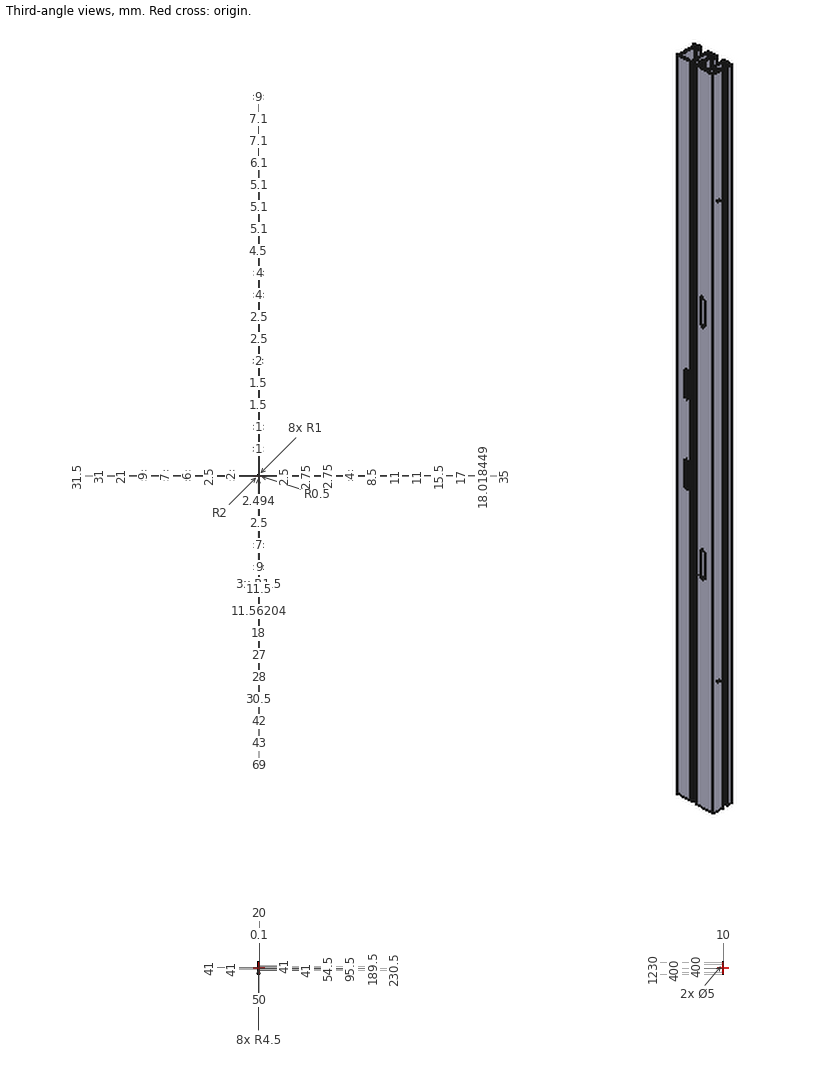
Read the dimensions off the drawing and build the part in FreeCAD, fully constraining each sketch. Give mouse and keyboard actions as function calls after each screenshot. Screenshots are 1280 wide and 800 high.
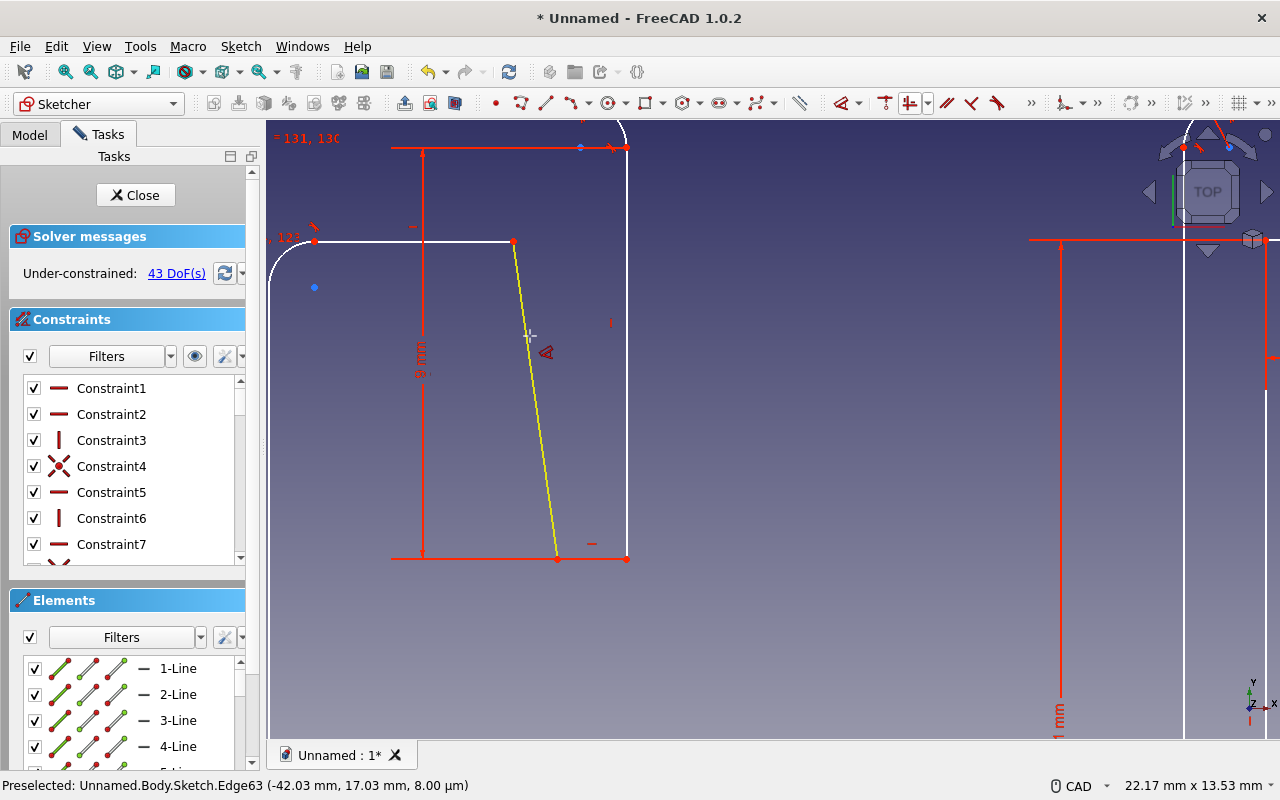
click(526, 337)
click(535, 208)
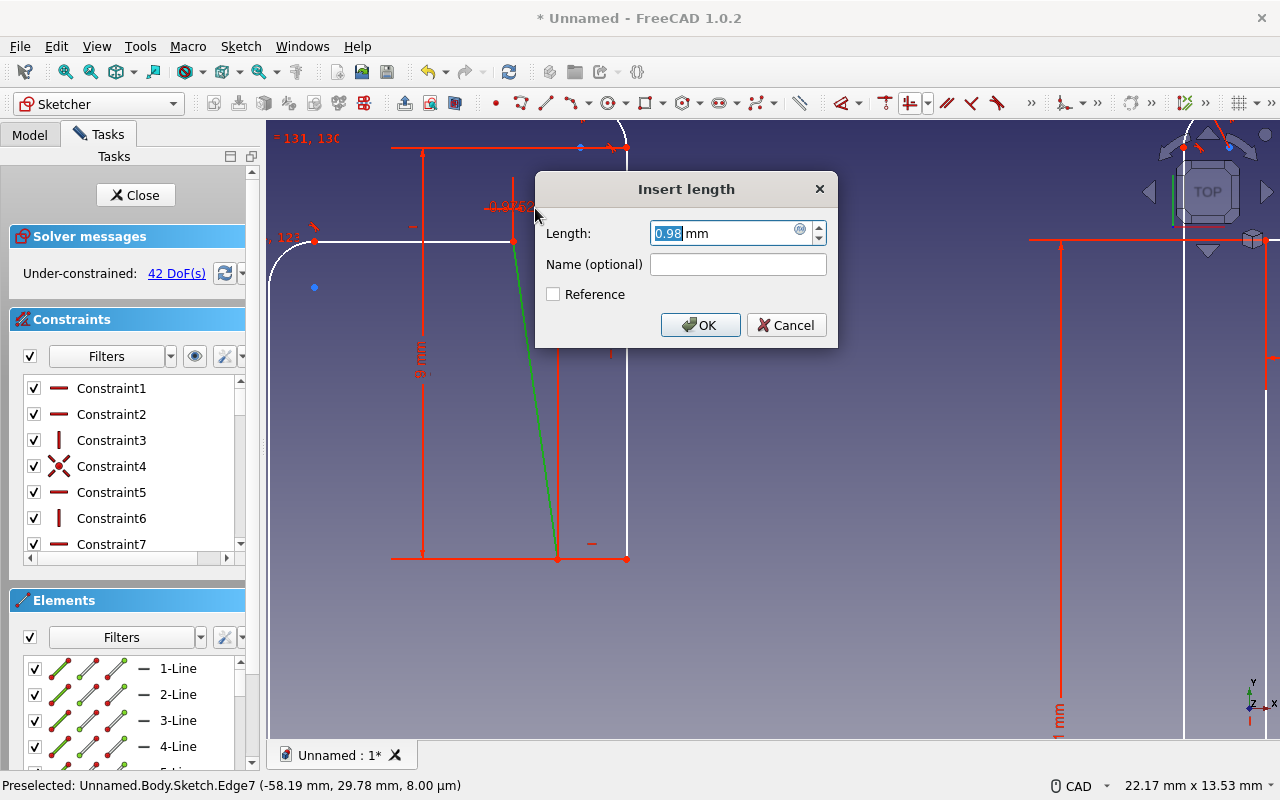
text(1)
key(Return)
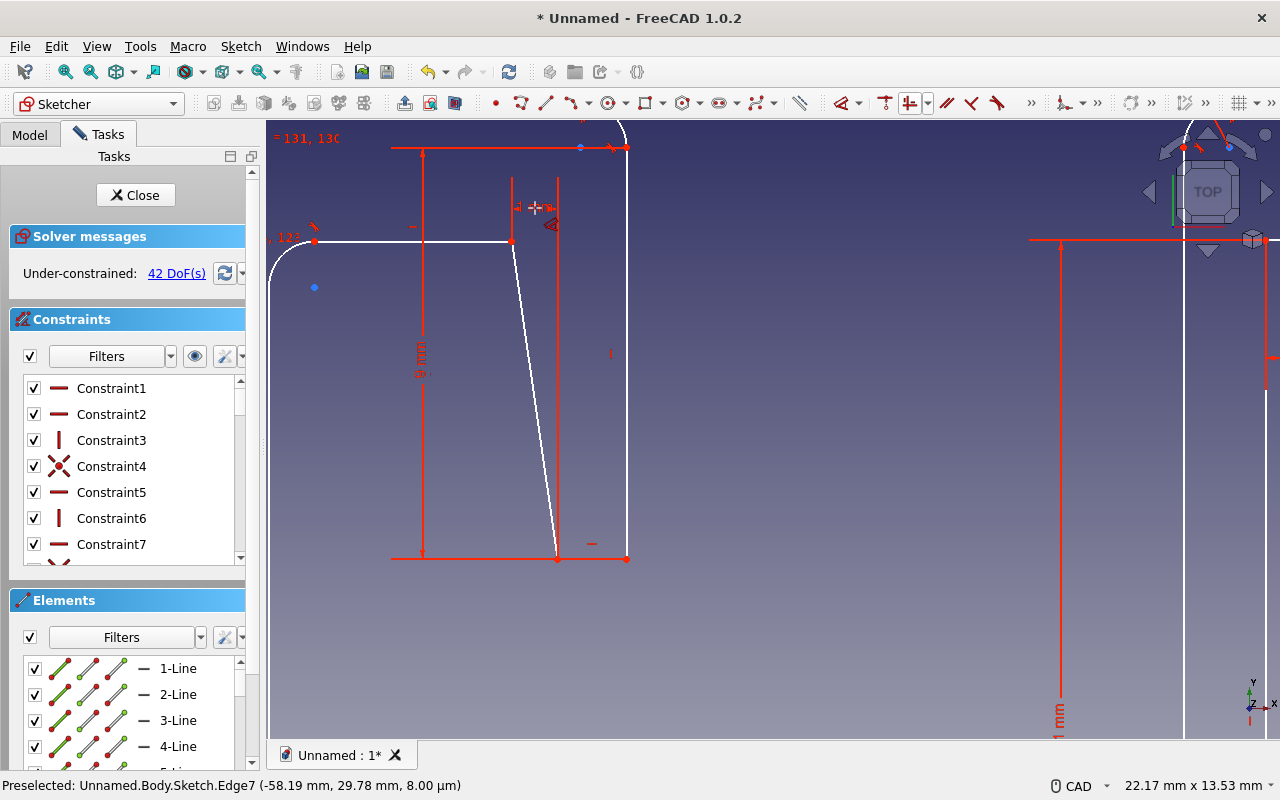
scroll(530, 336, down, 9)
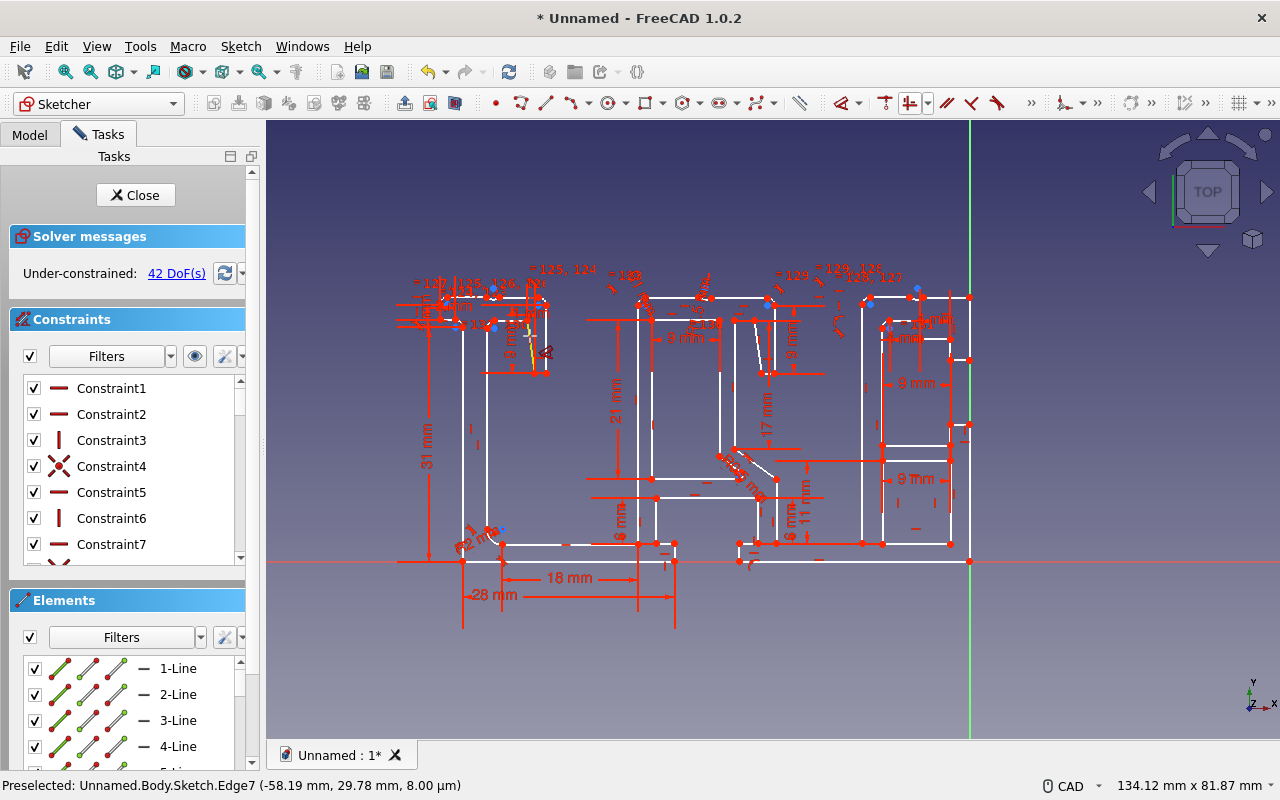
click(530, 336)
click(569, 365)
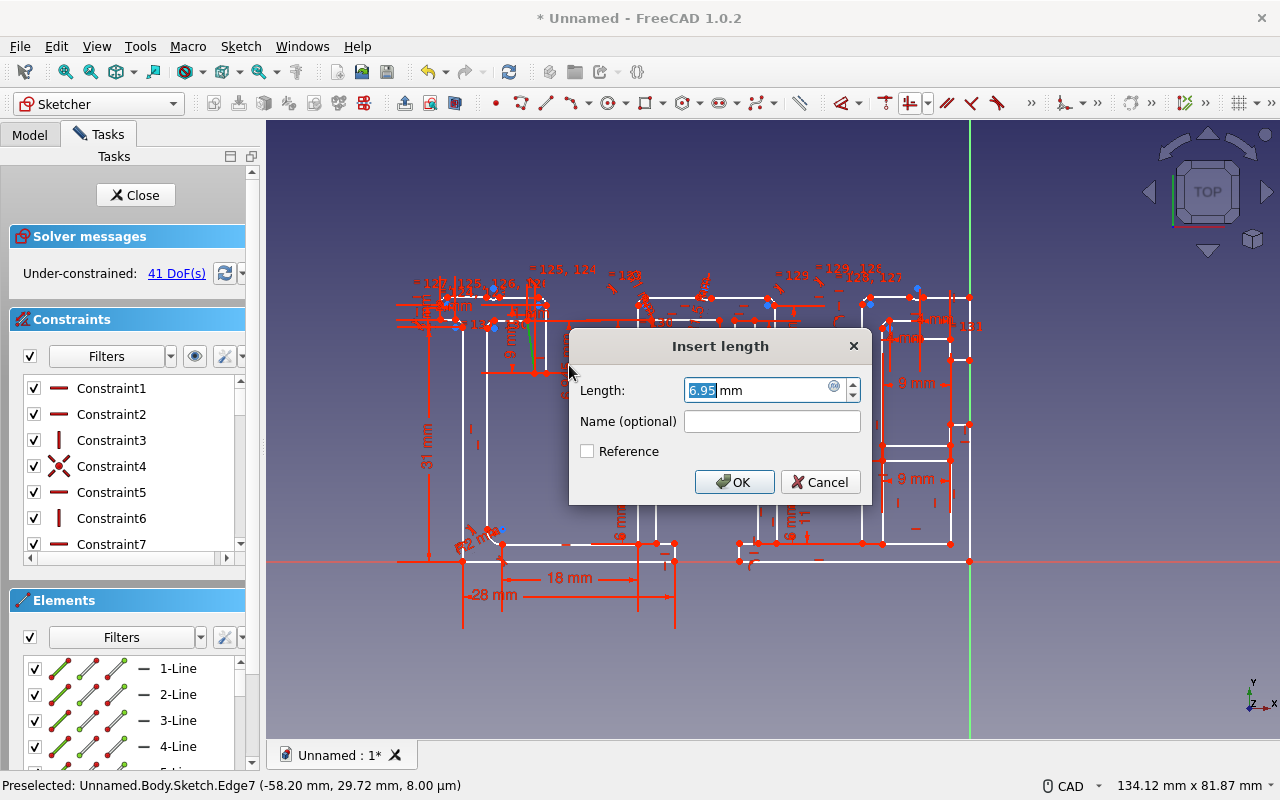
text(7)
key(Return)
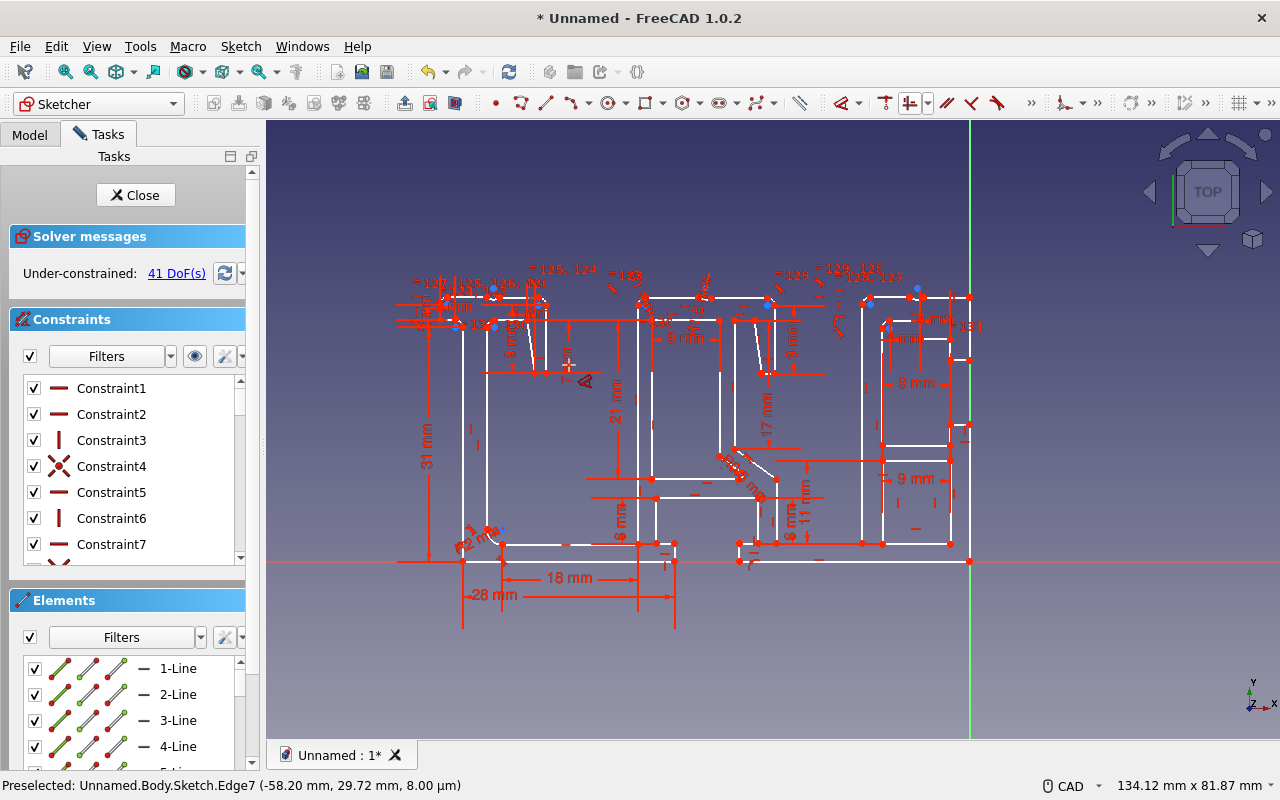
scroll(764, 470, up, 2)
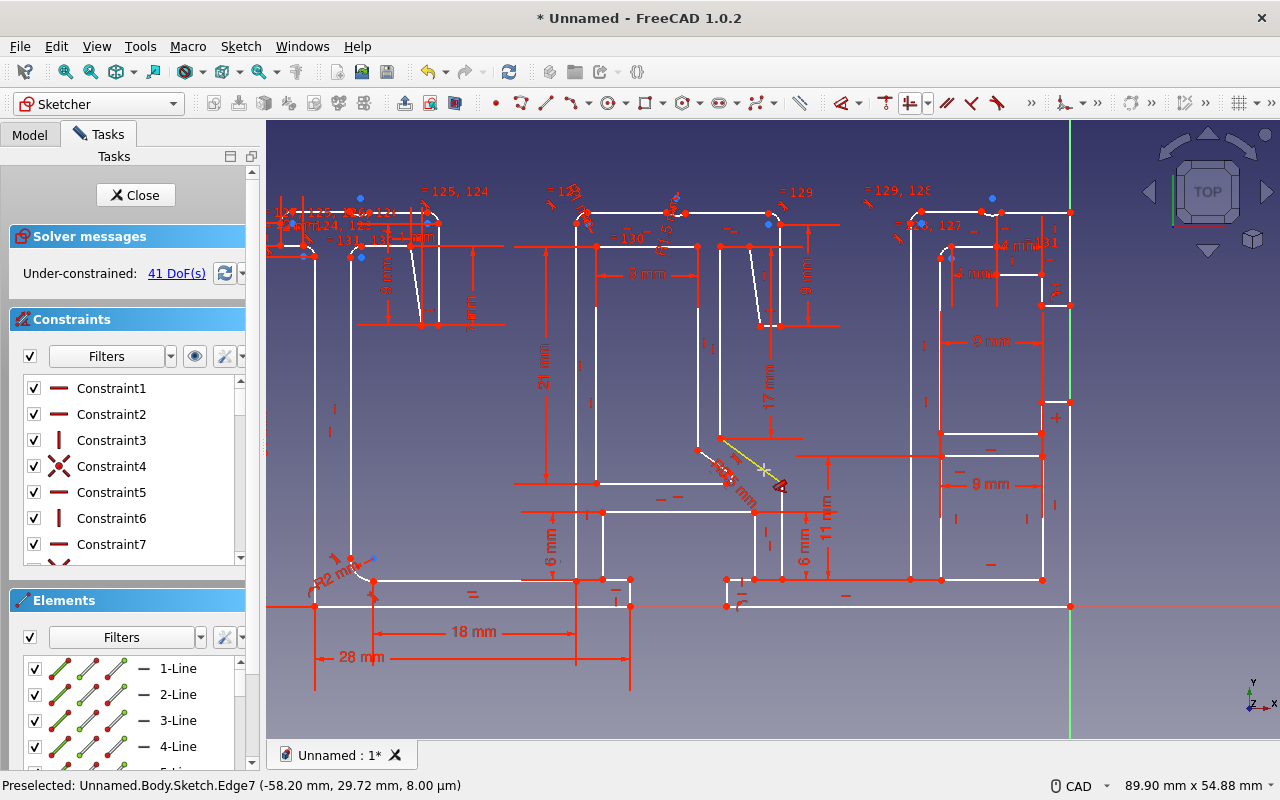
click(764, 470)
click(816, 461)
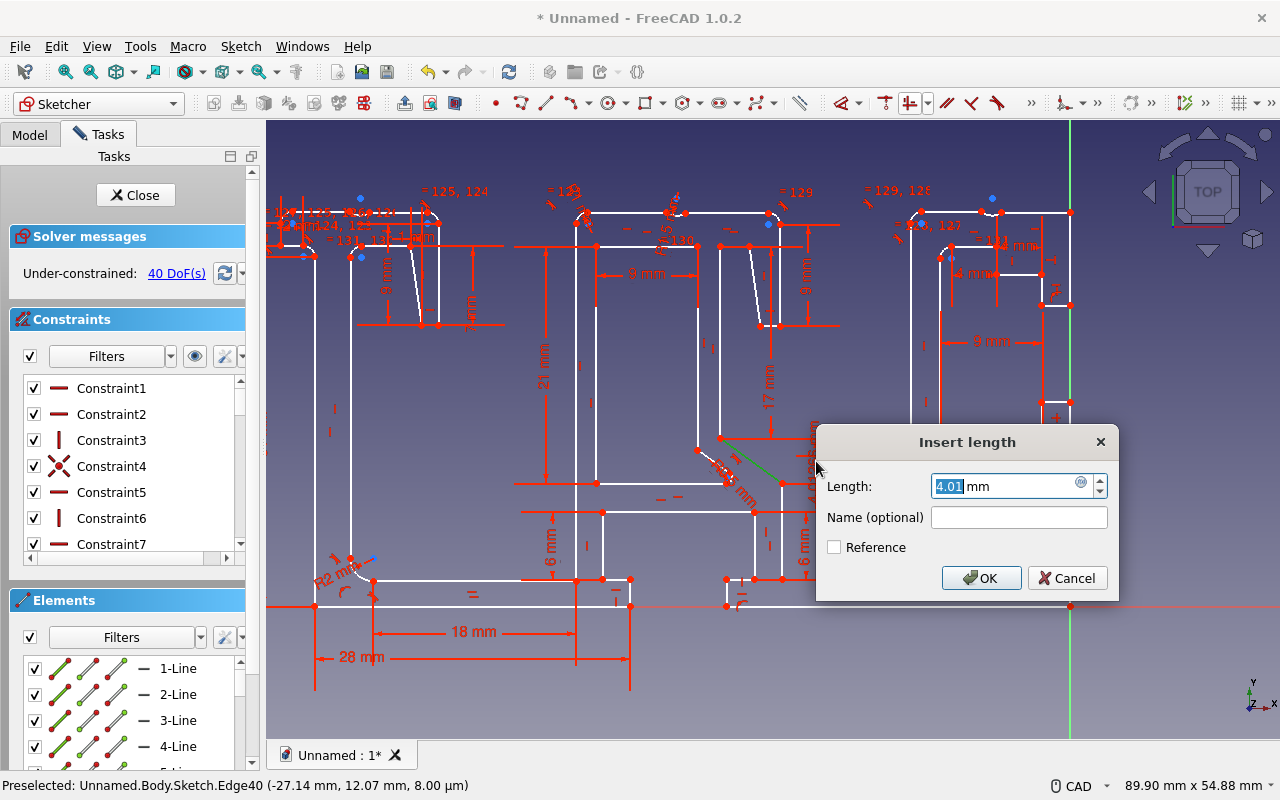
text(4)
key(Return)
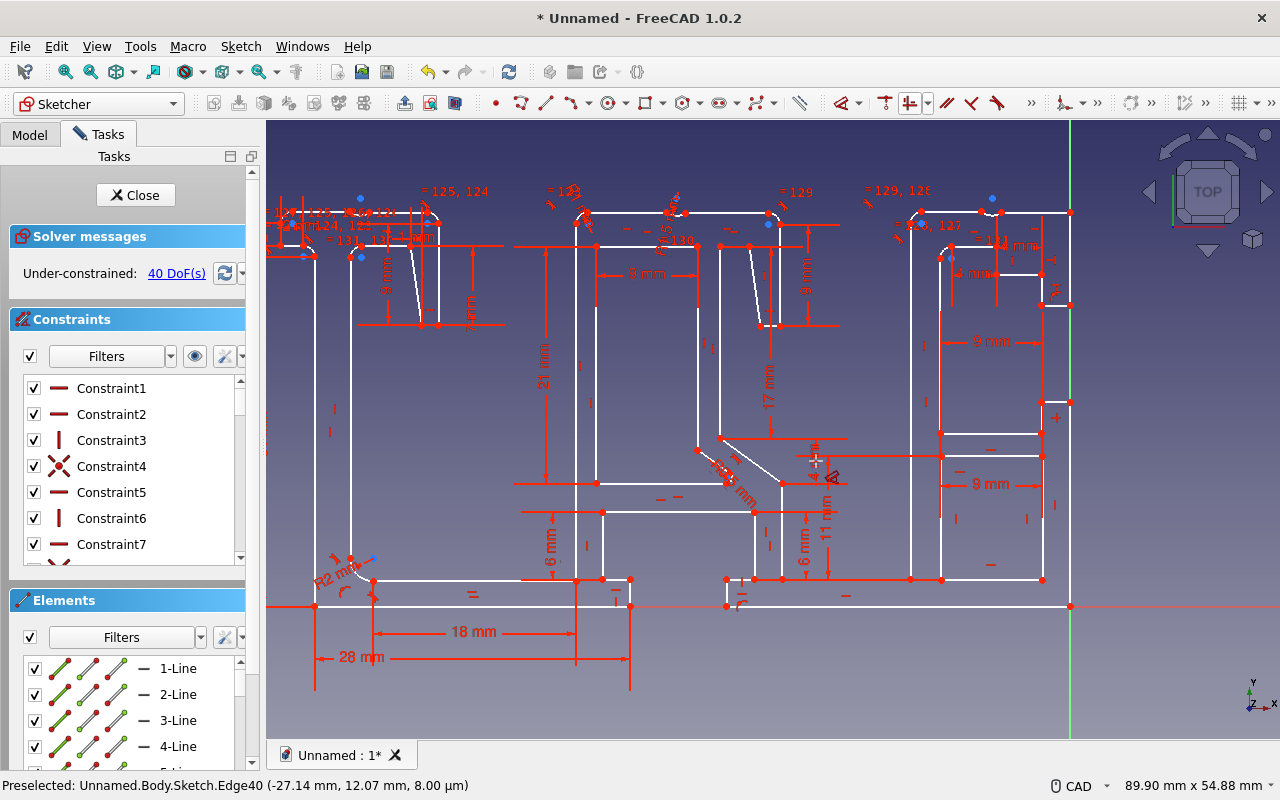
scroll(753, 271, up, 7)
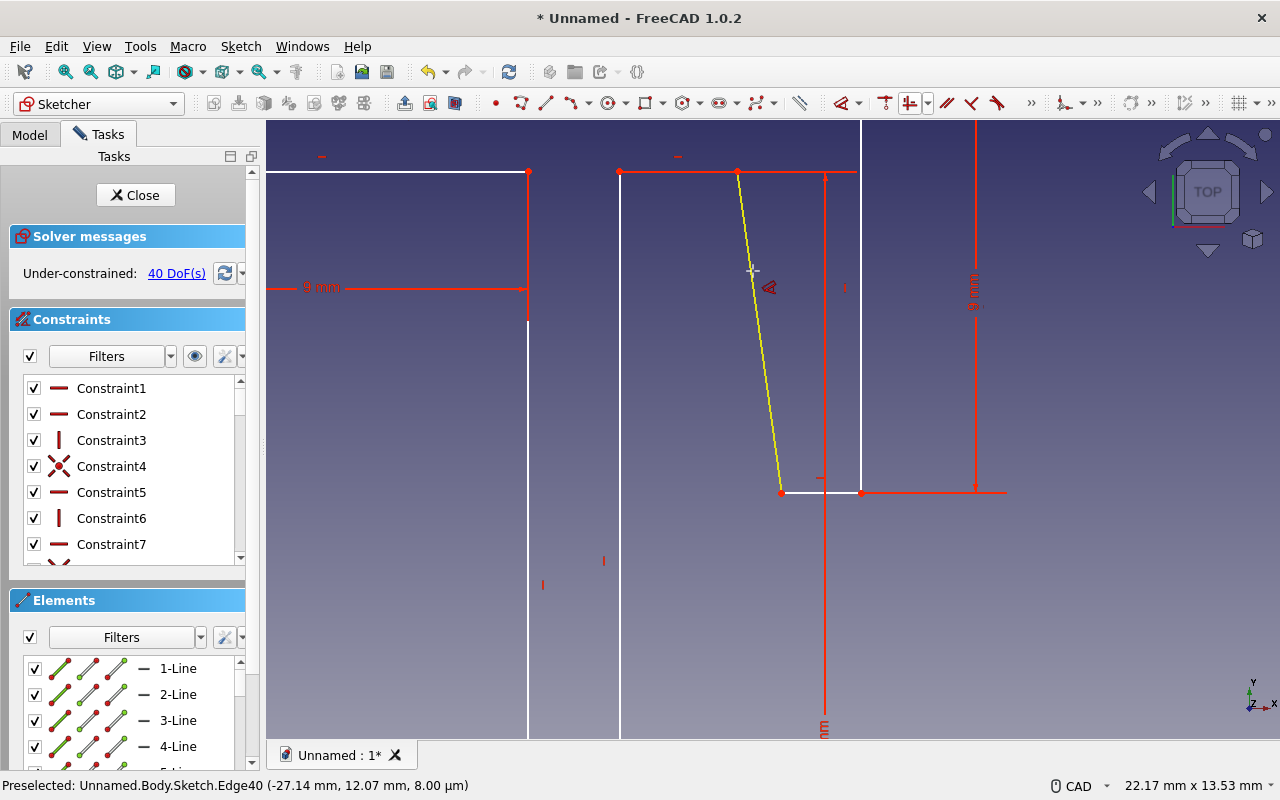
click(751, 268)
click(760, 527)